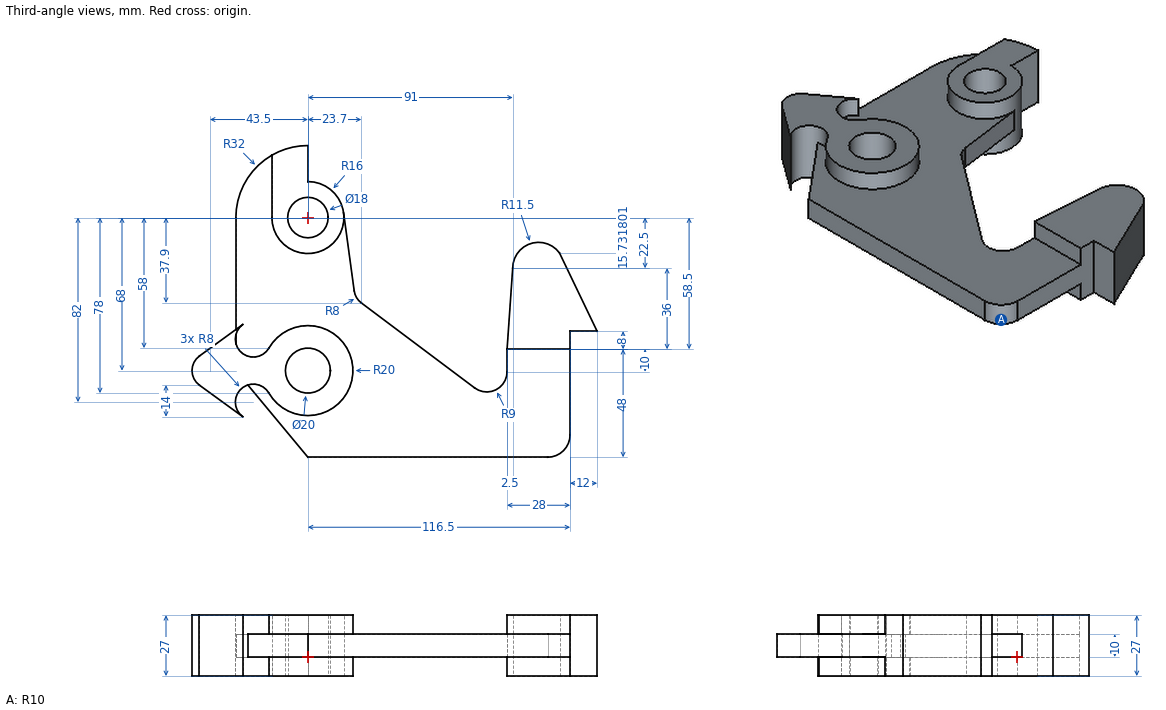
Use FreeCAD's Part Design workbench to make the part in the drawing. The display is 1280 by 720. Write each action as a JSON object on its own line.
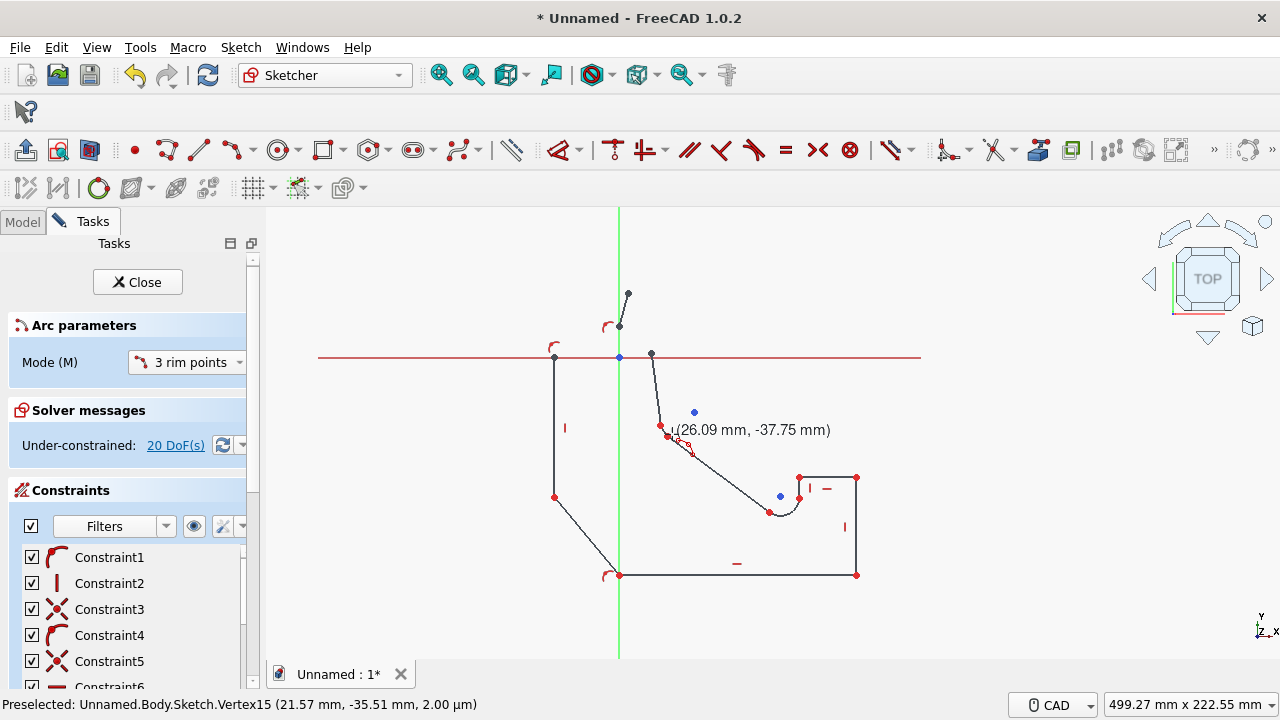
{"action": "scroll", "coordinate": [652, 354], "scroll_direction": "up", "scroll_amount": 7}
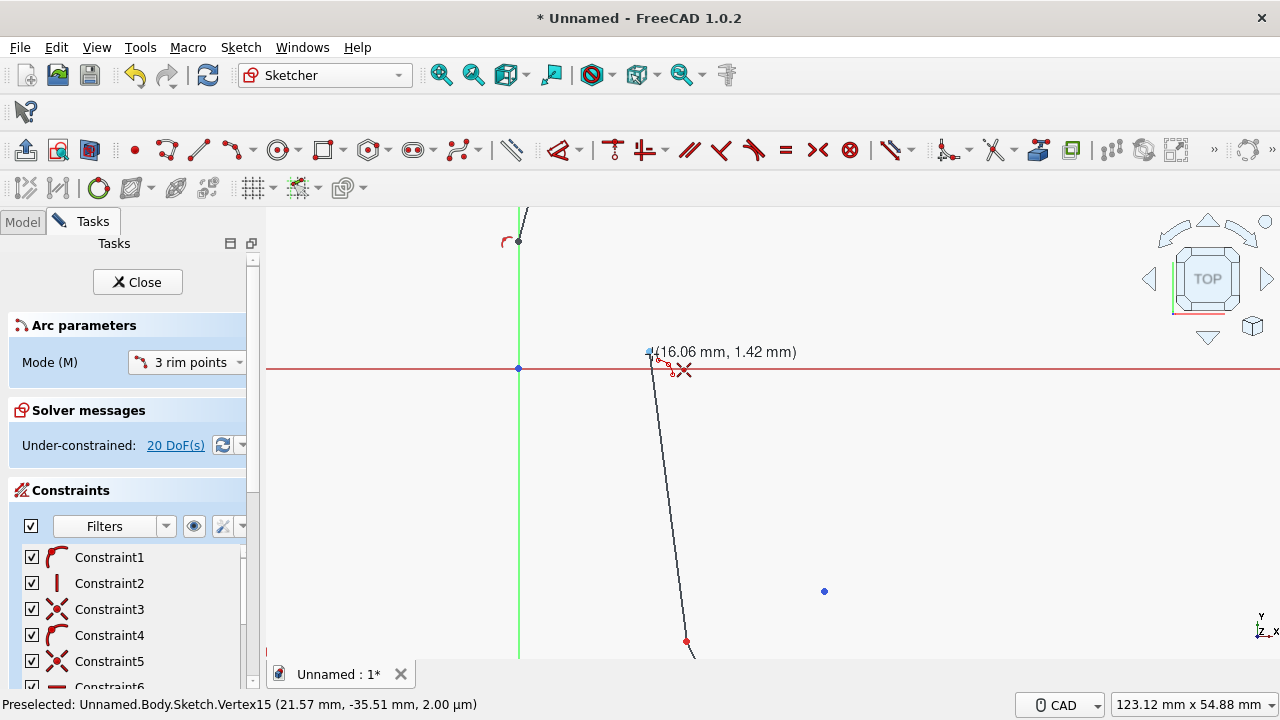
{"action": "left_click", "coordinate": [650, 352]}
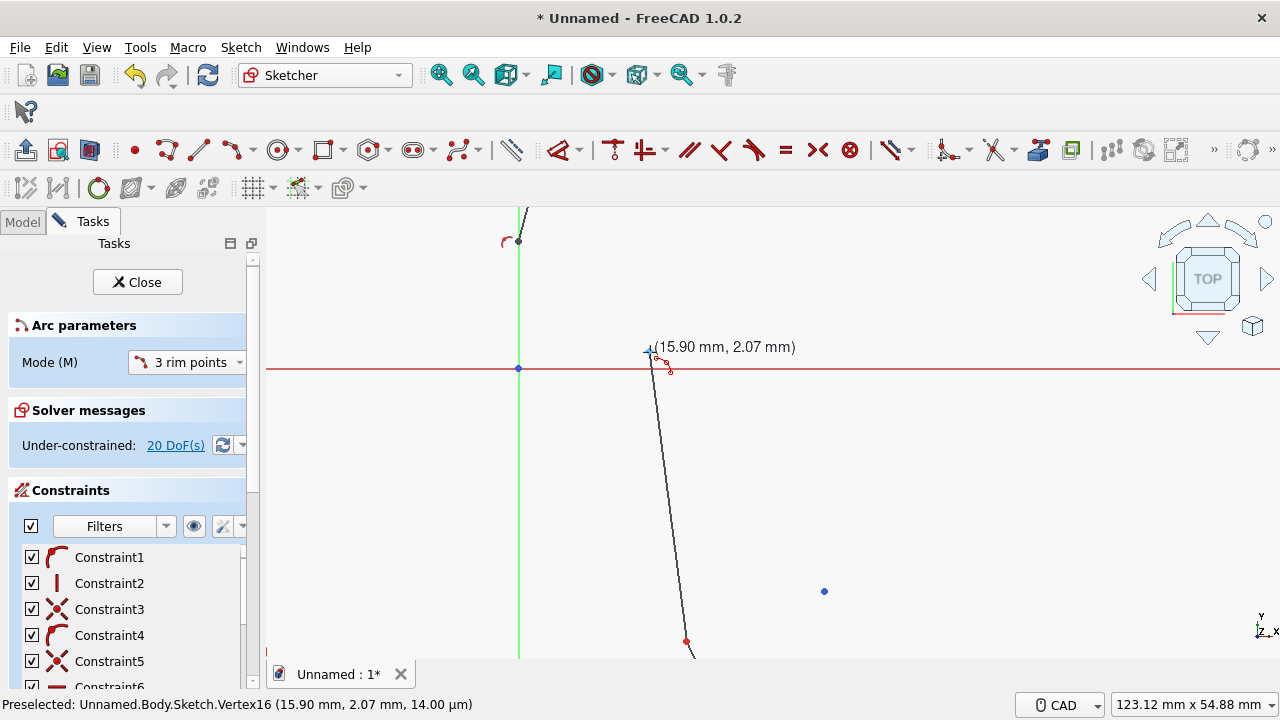
{"action": "scroll", "coordinate": [651, 354], "scroll_direction": "down", "scroll_amount": 7}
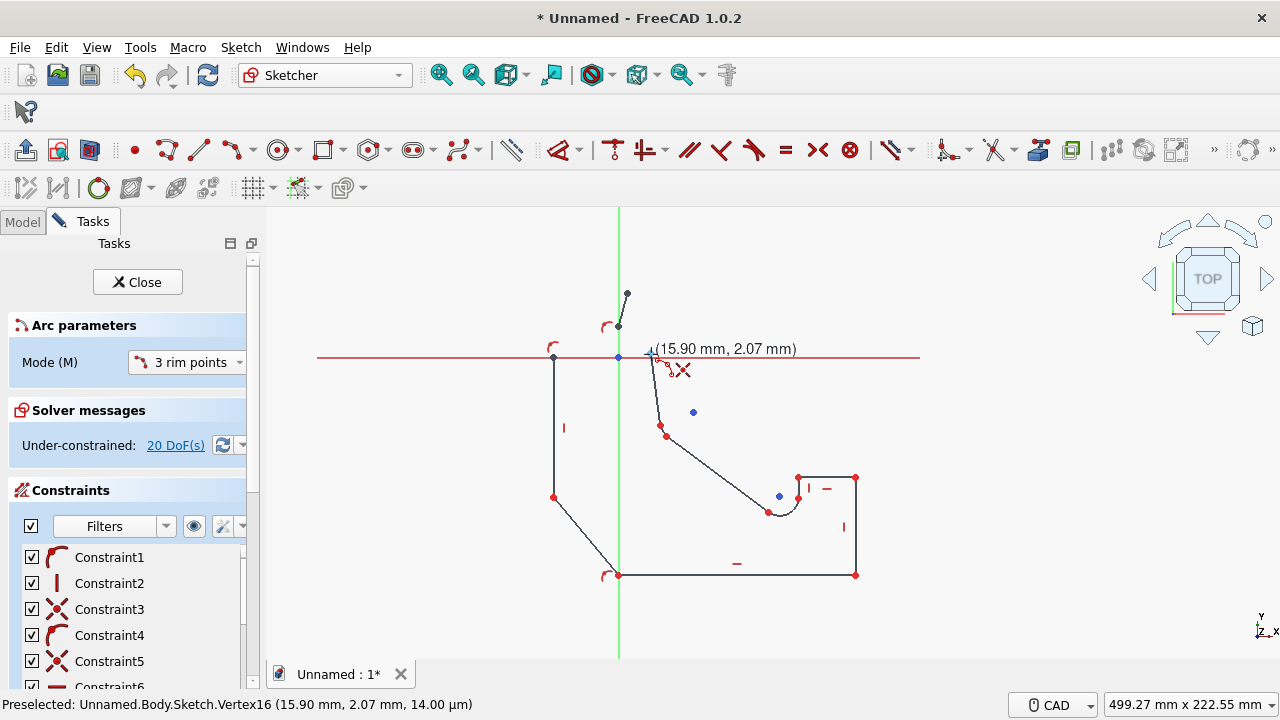
{"action": "left_click", "coordinate": [619, 326]}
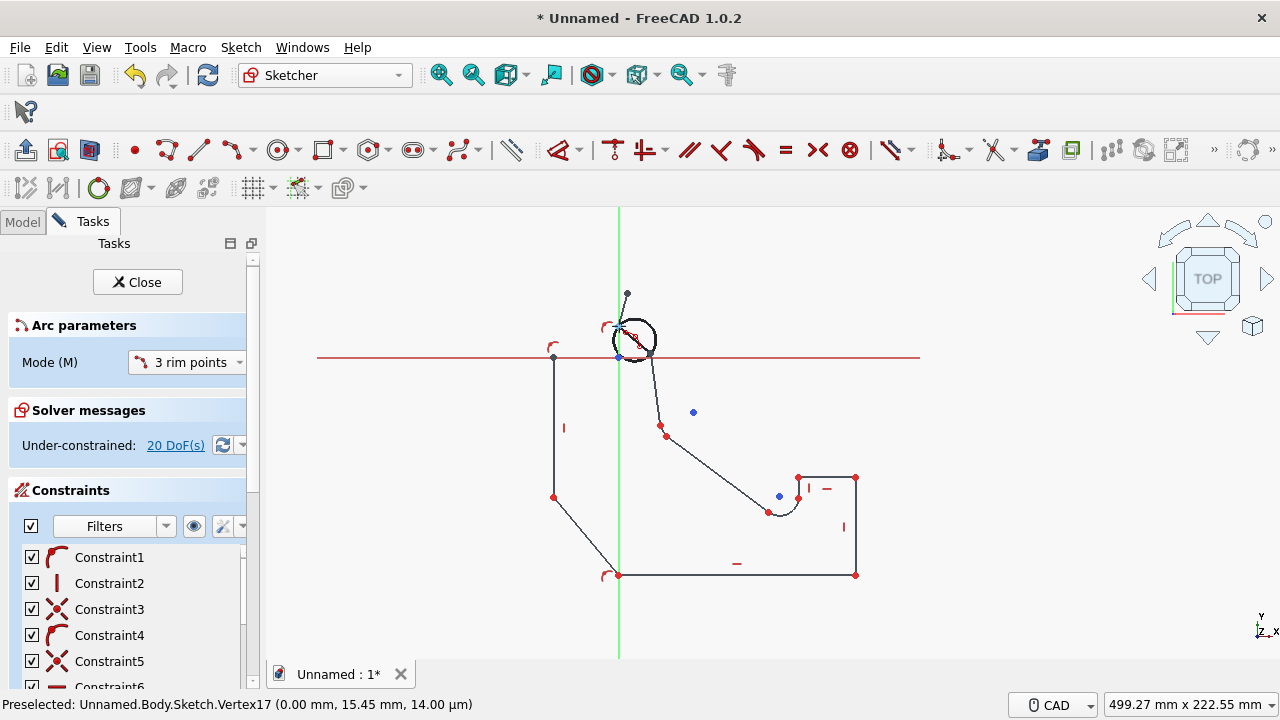
{"action": "scroll", "coordinate": [640, 333], "scroll_direction": "up", "scroll_amount": 4}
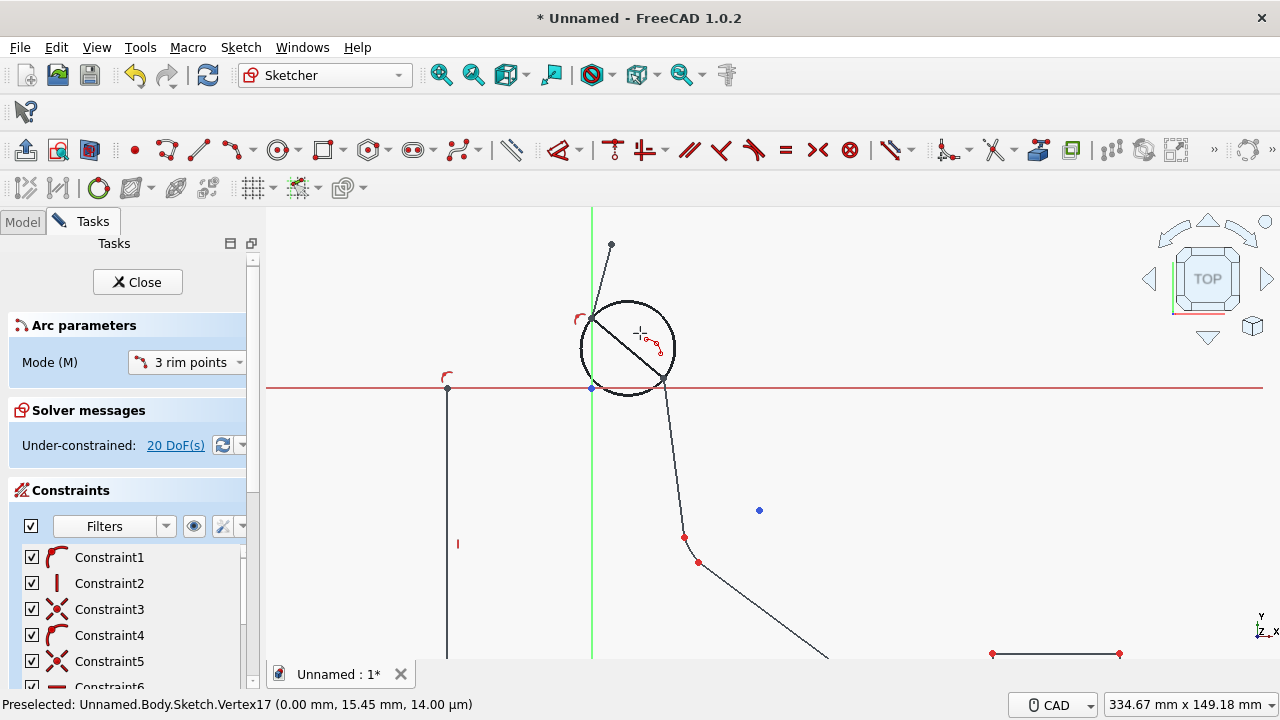
{"action": "left_click", "coordinate": [640, 334]}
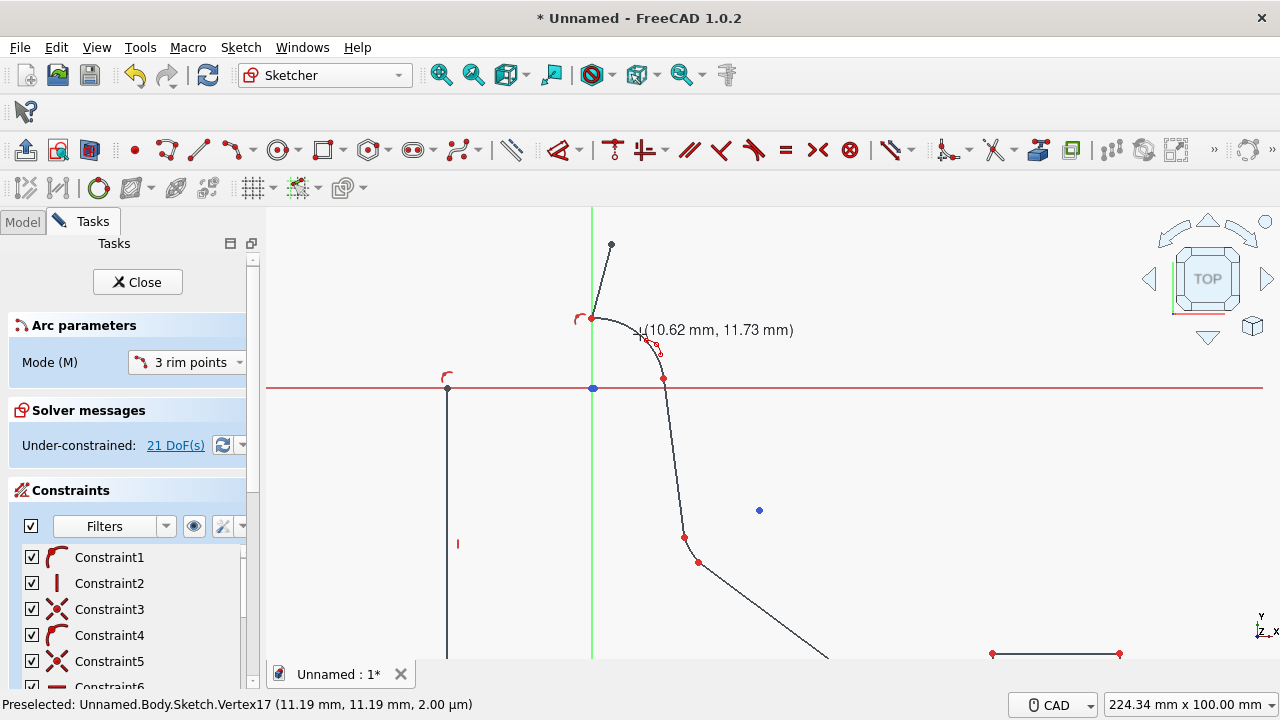
{"action": "left_click", "coordinate": [611, 245]}
{"action": "left_click", "coordinate": [447, 388]}
{"action": "left_click", "coordinate": [490, 286]}
{"action": "key", "text": "Escape"}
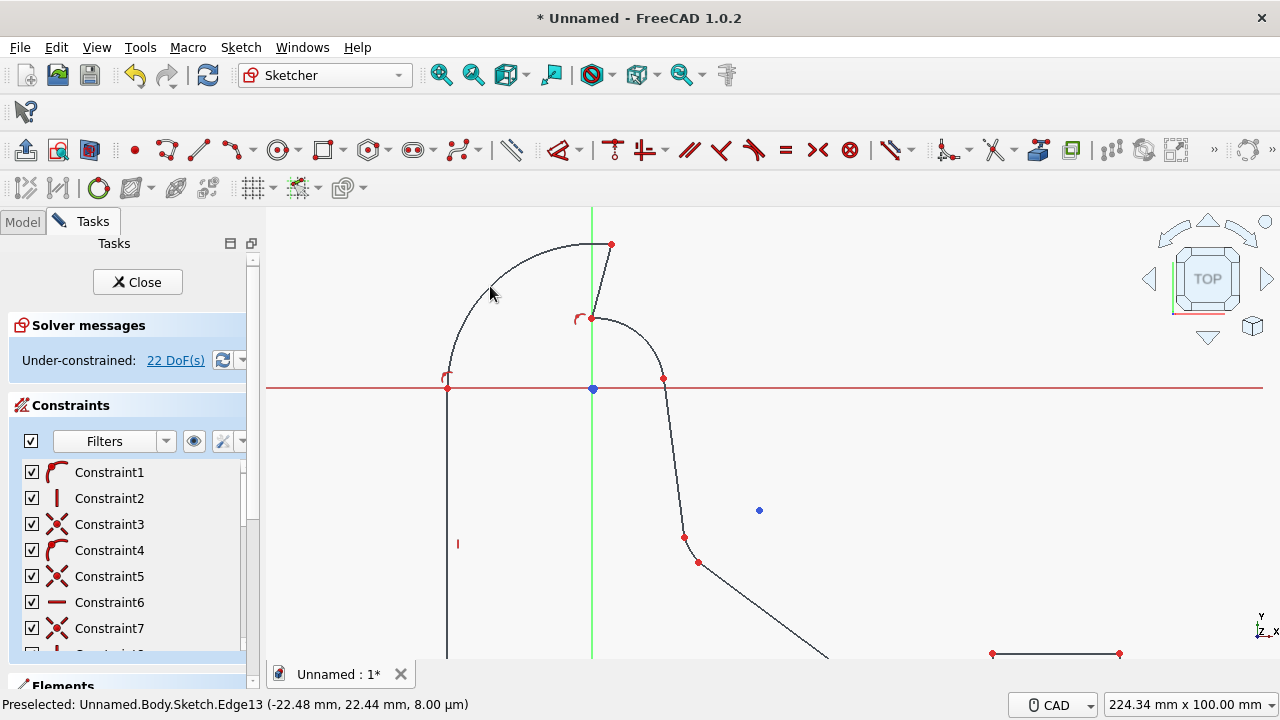
{"action": "scroll", "coordinate": [640, 332], "scroll_direction": "down", "scroll_amount": 4}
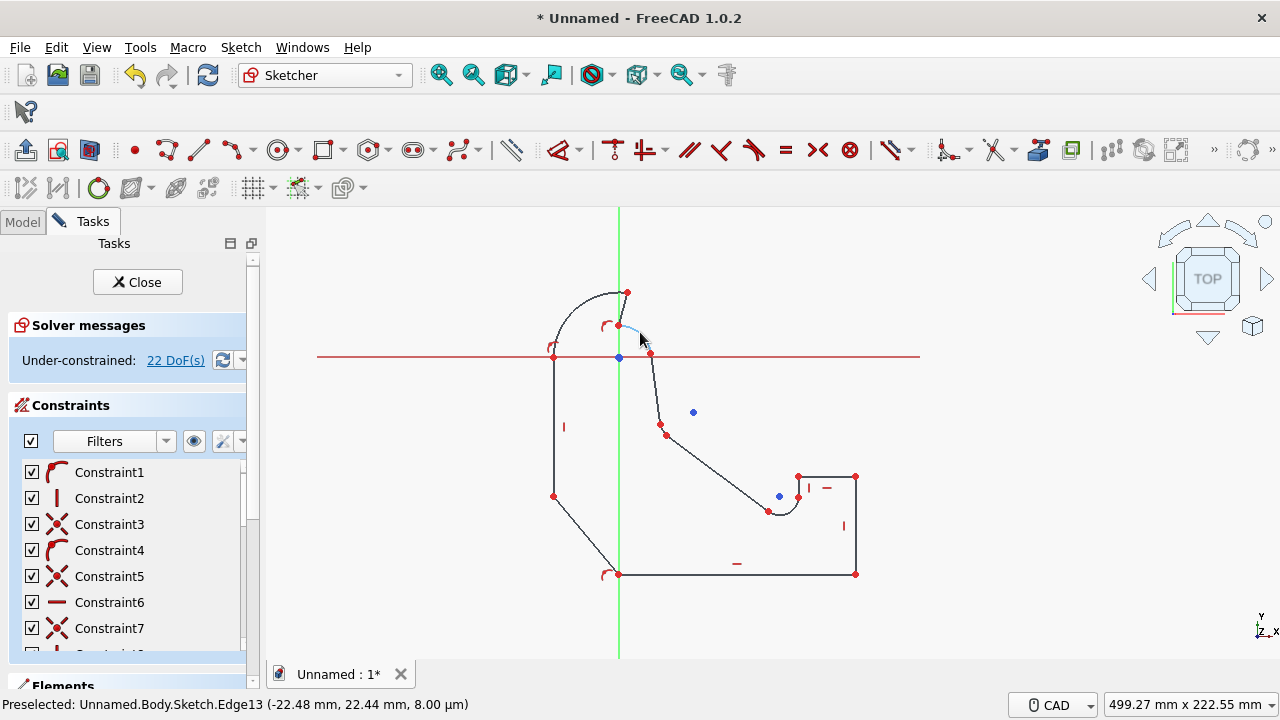
{"action": "scroll", "coordinate": [799, 483], "scroll_direction": "up", "scroll_amount": 4}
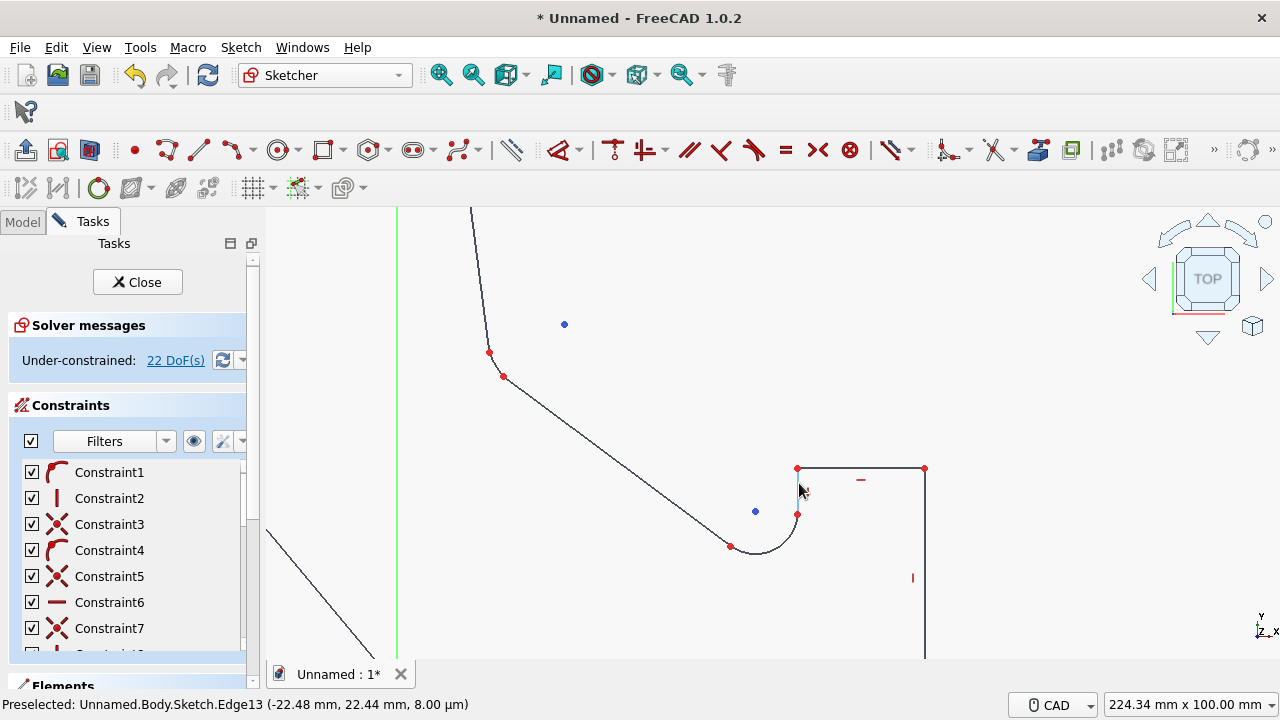
{"action": "left_click", "coordinate": [798, 482]}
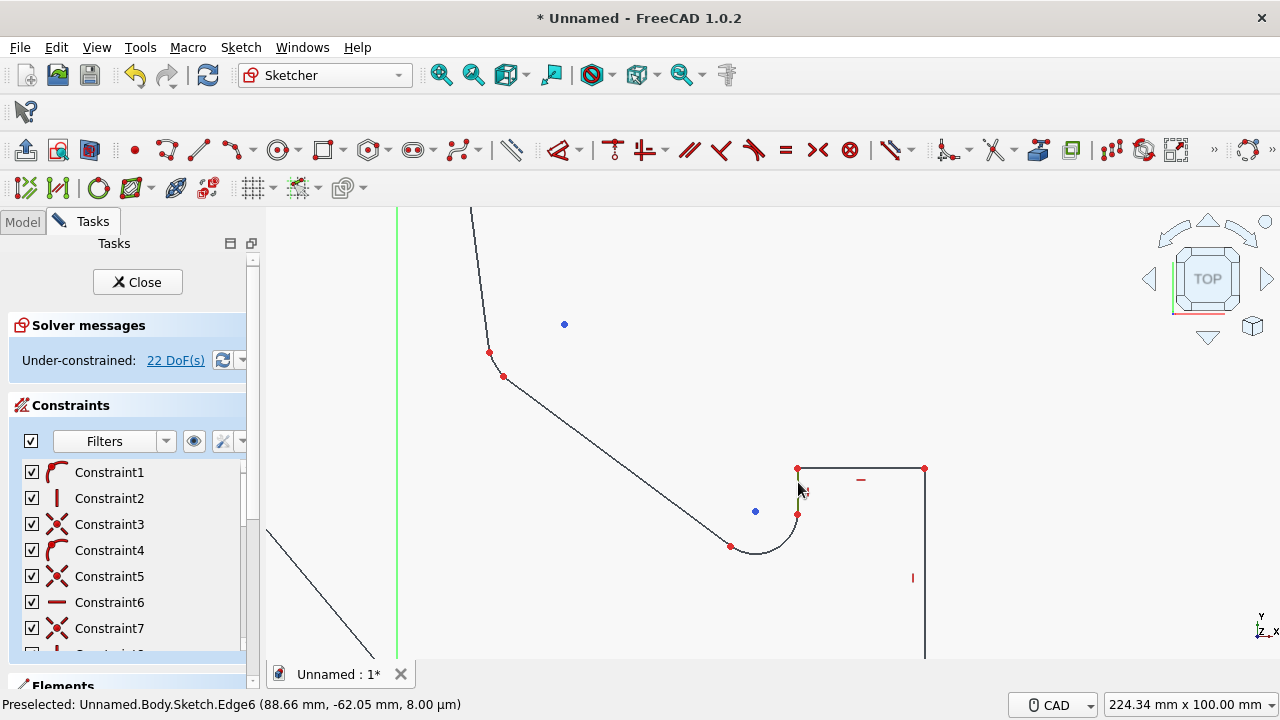
{"action": "left_click", "coordinate": [756, 554]}